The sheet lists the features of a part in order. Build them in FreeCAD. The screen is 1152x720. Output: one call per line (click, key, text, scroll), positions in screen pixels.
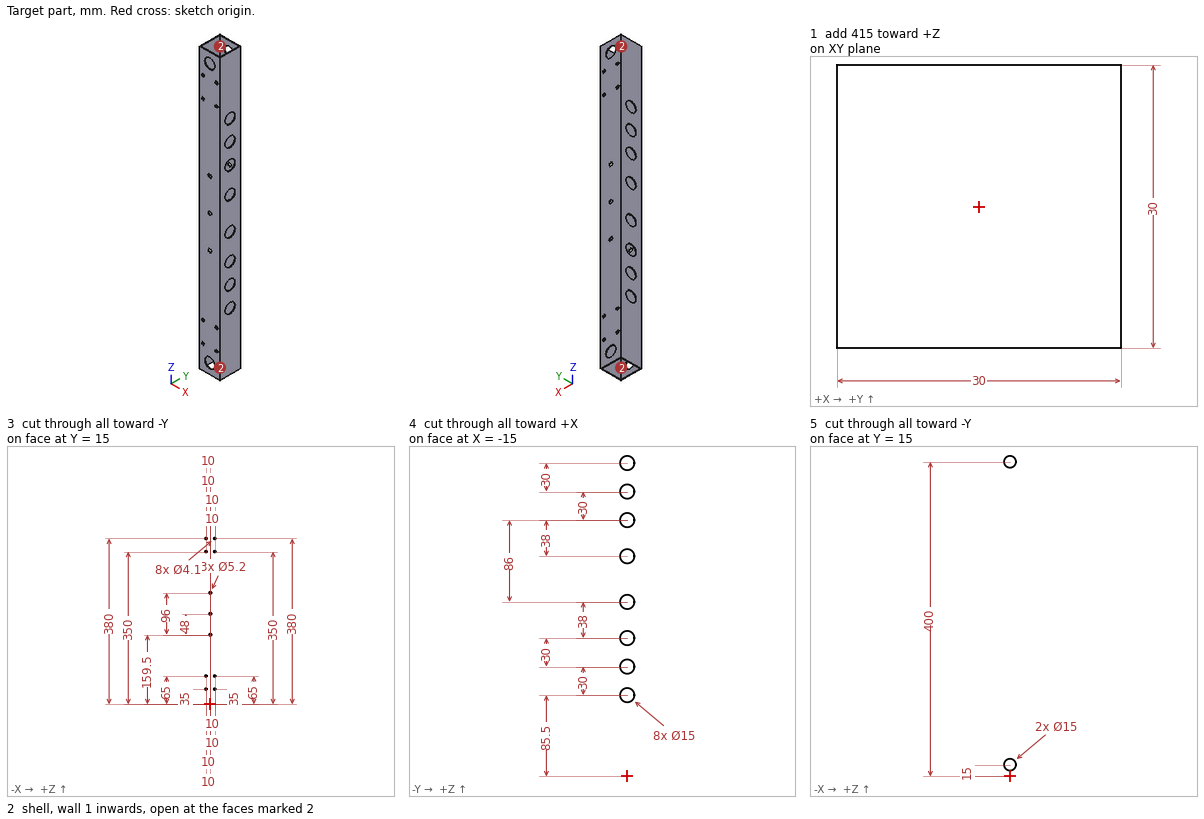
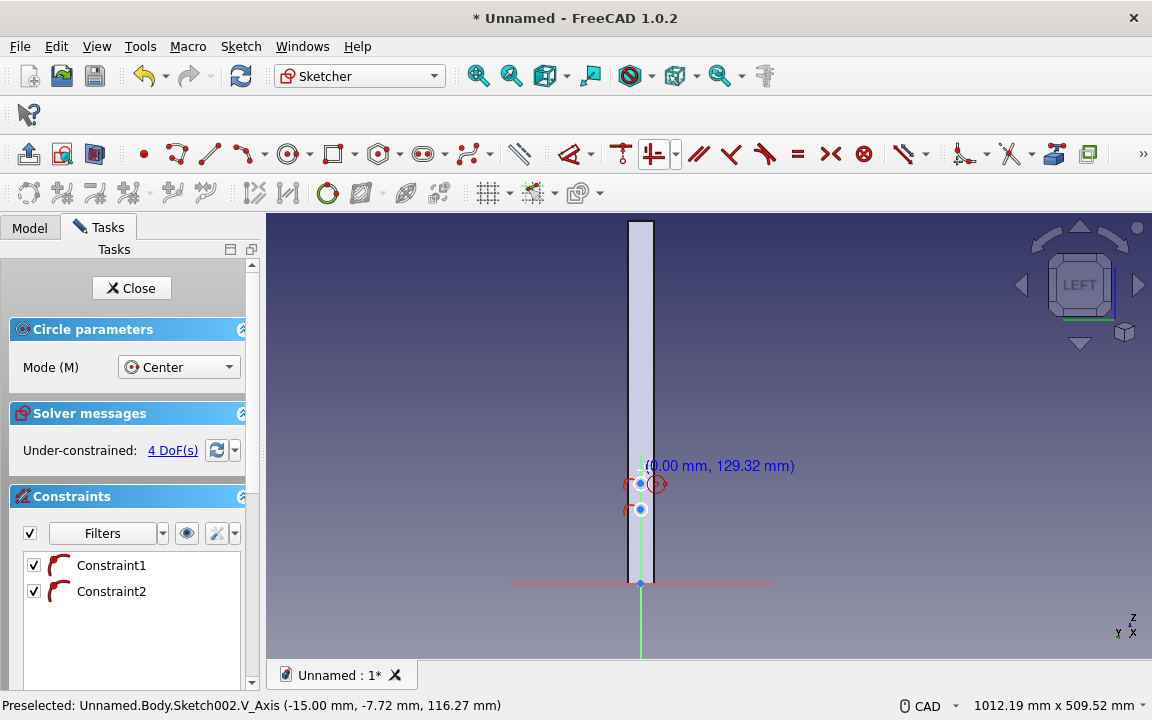
click(641, 457)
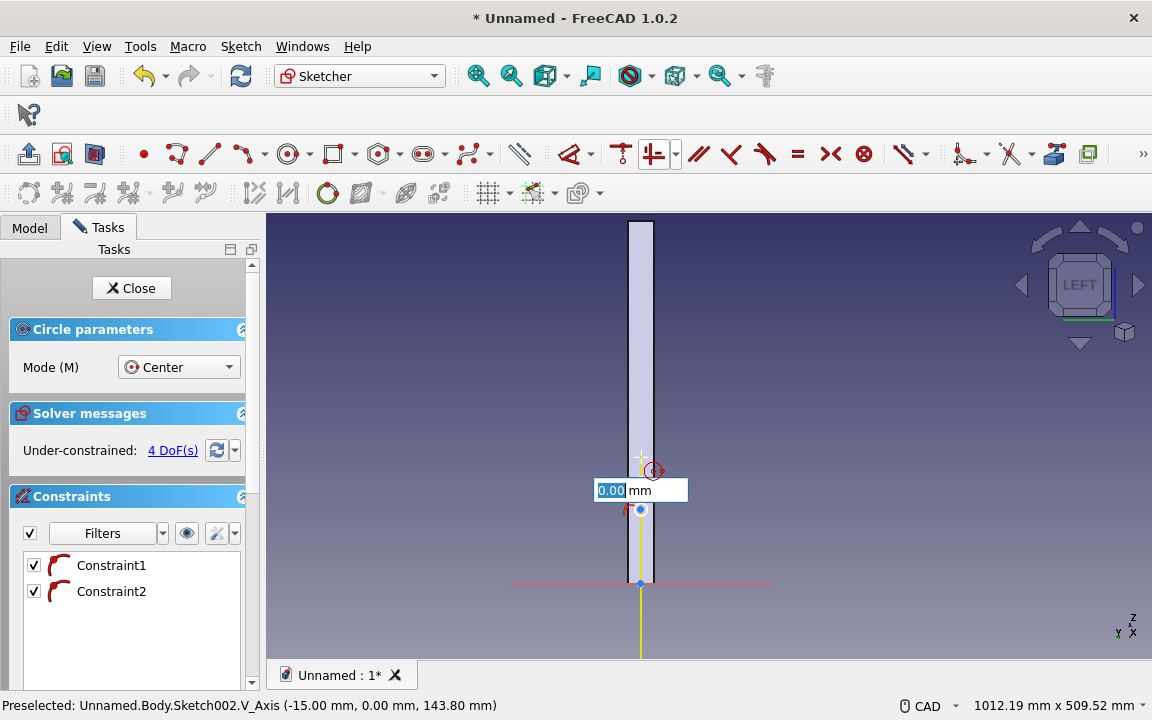
scroll(647, 454, up, 5)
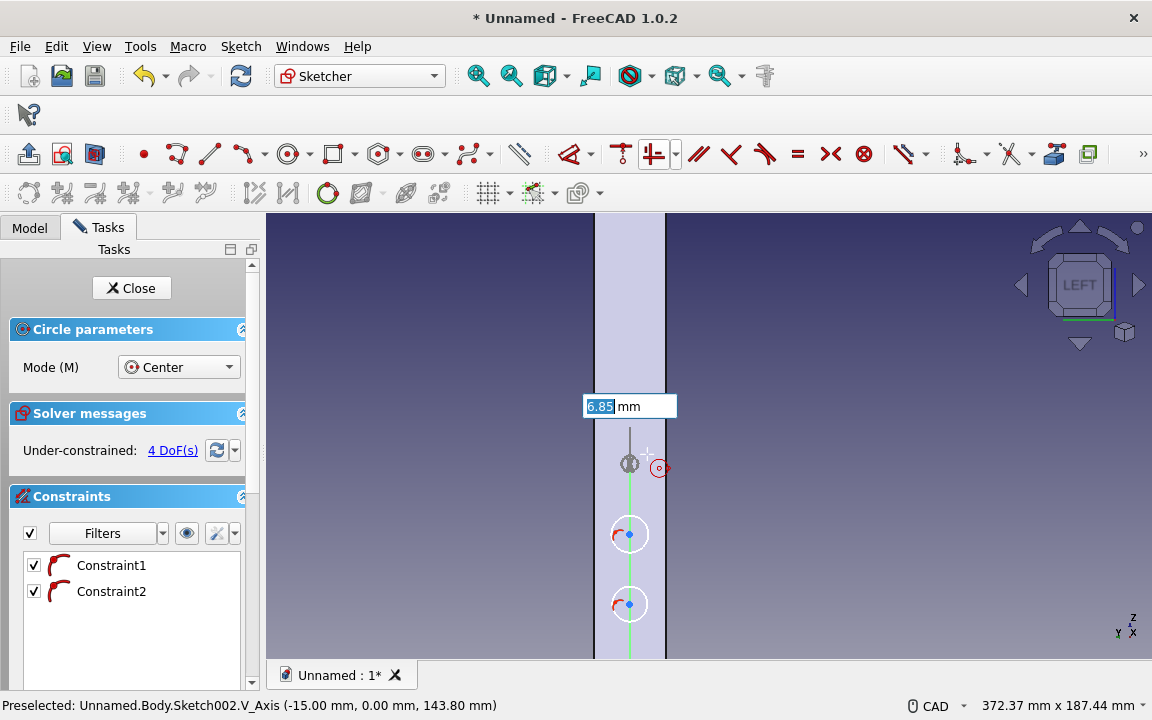
click(647, 454)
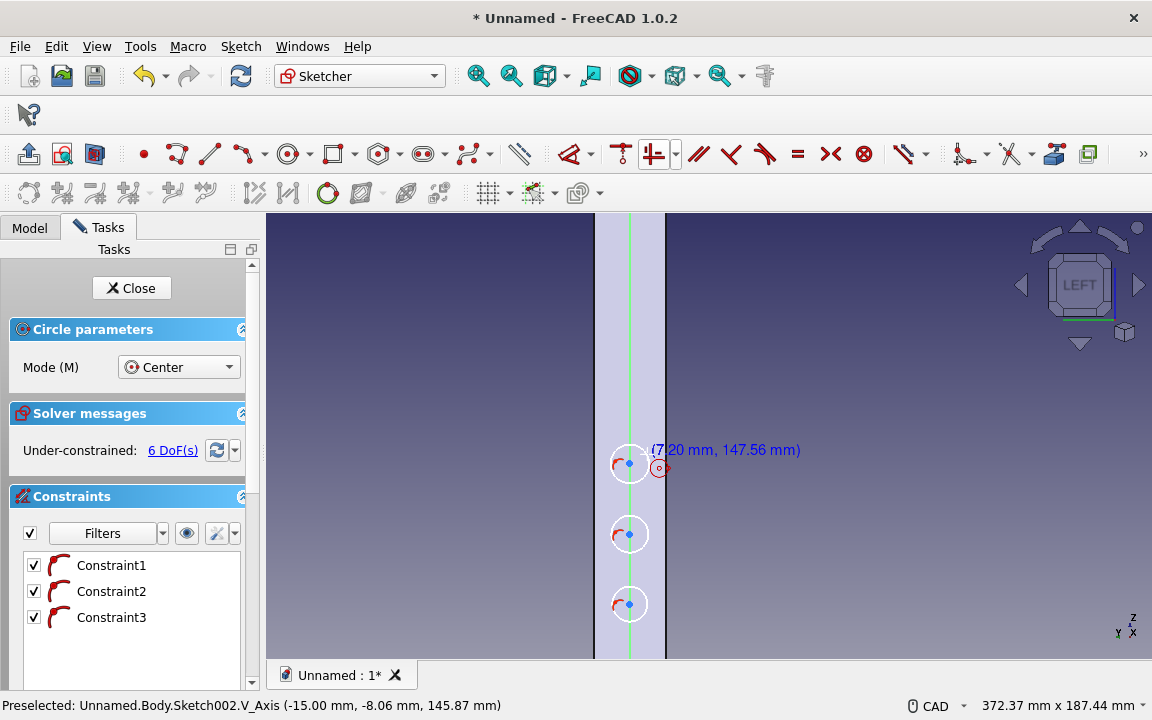
scroll(647, 454, down, 5)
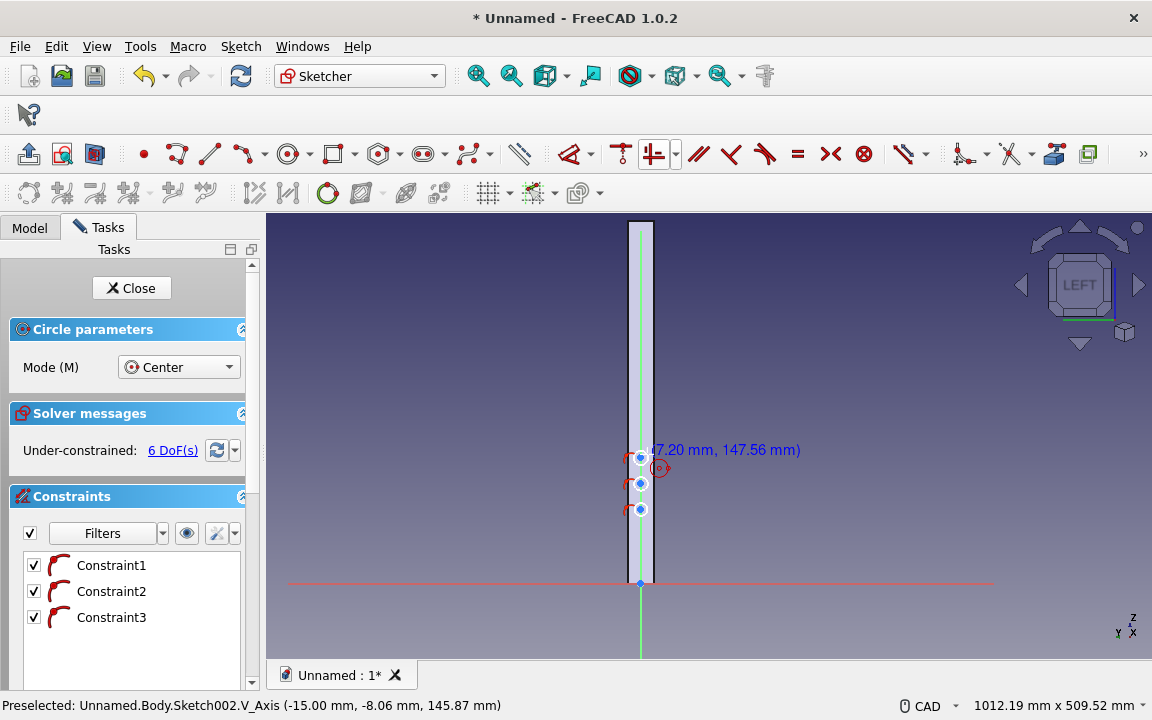
scroll(641, 348, up, 7)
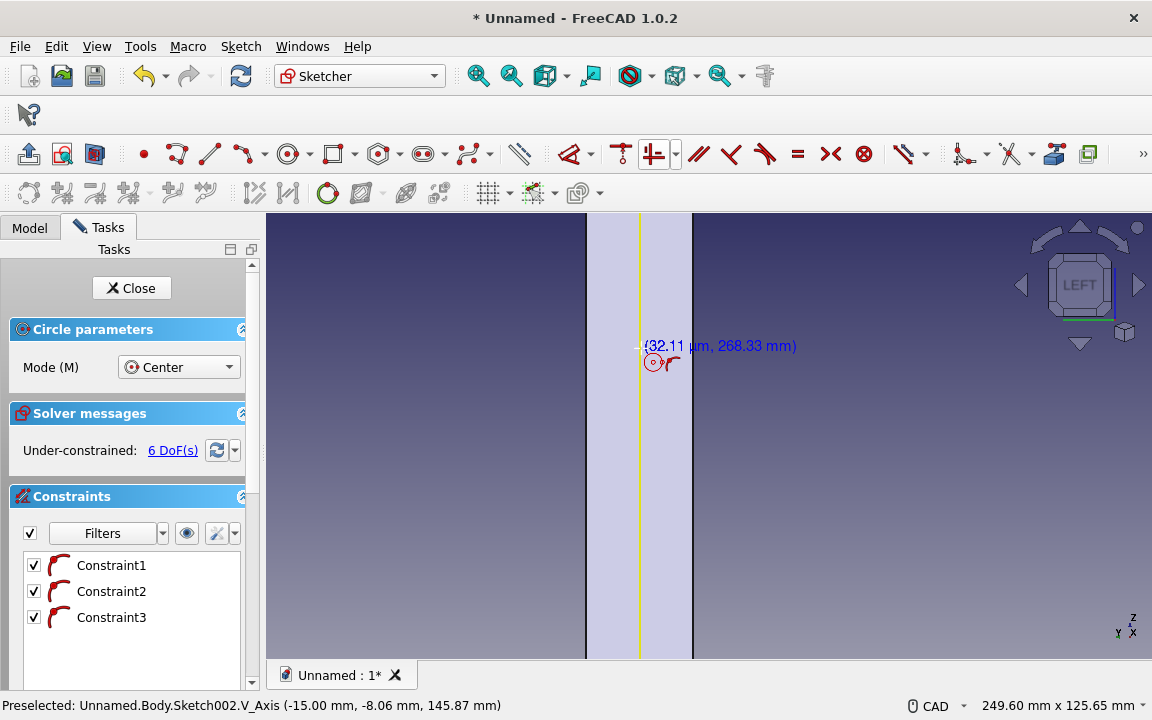
scroll(641, 348, down, 7)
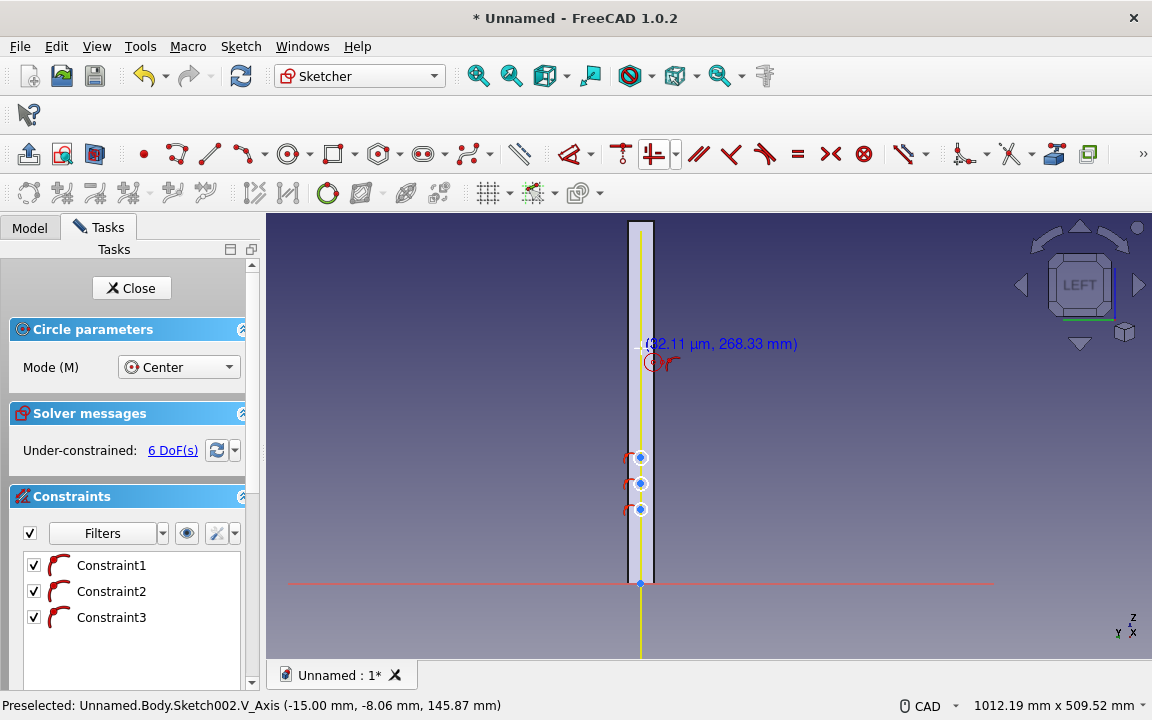
click(641, 348)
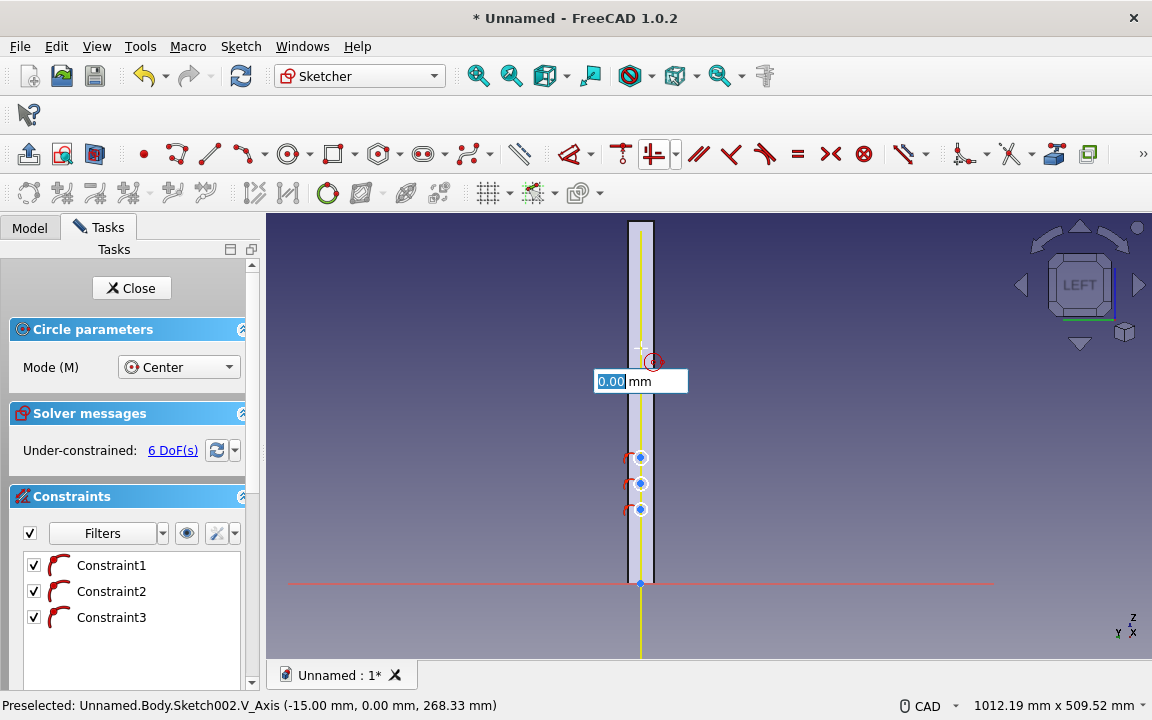
scroll(647, 346, up, 5)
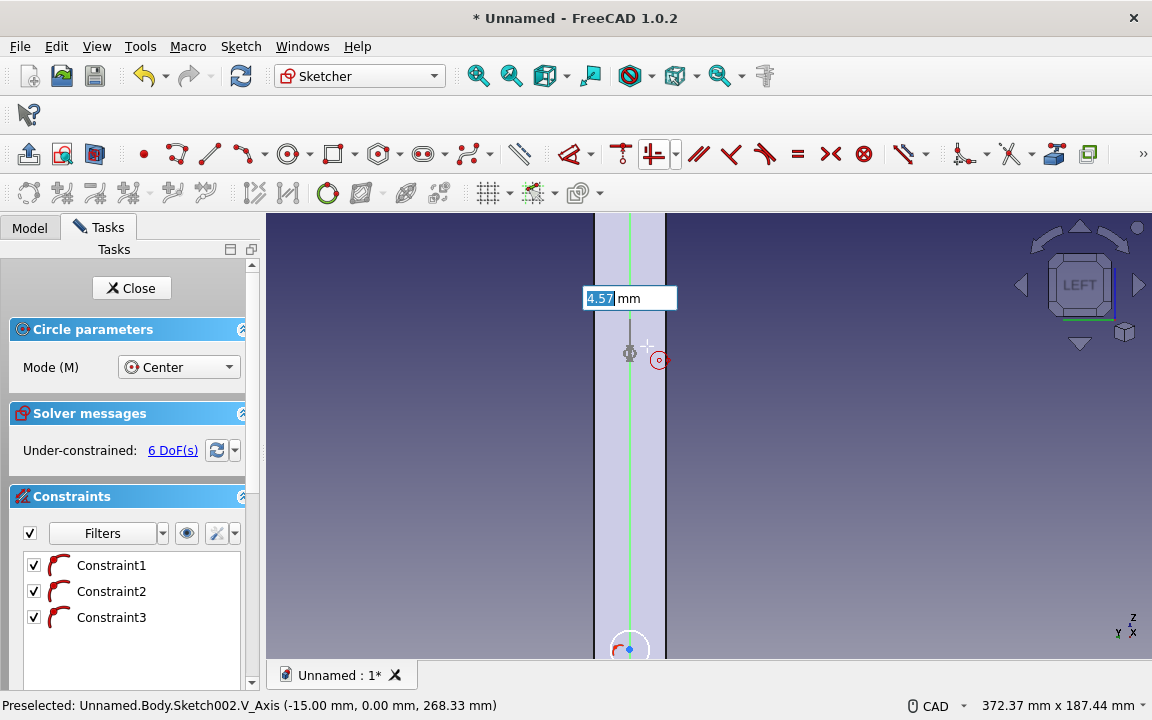
click(647, 345)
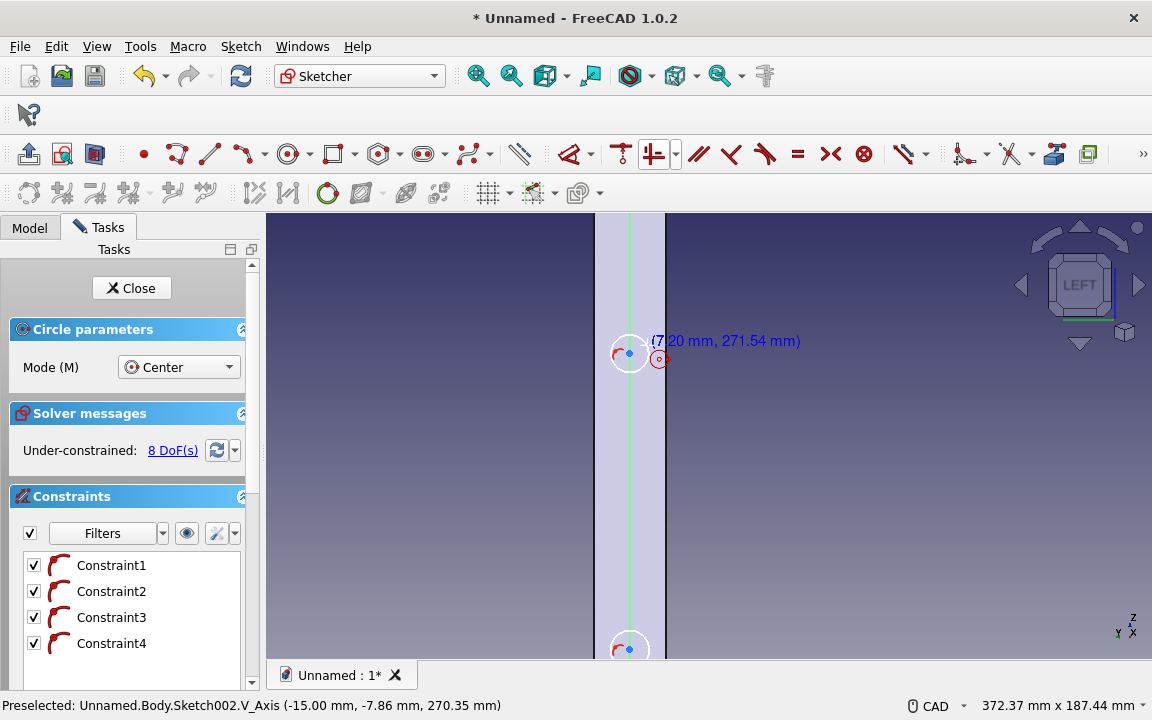
scroll(630, 279, up, 2)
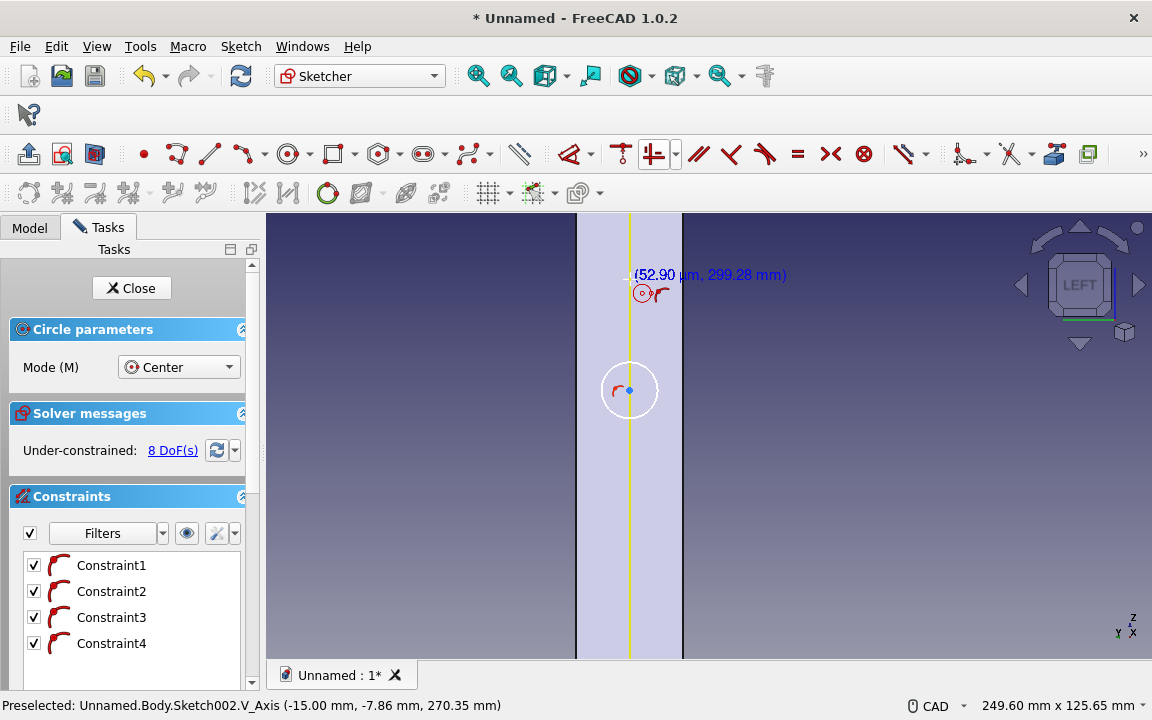
scroll(644, 335, down, 7)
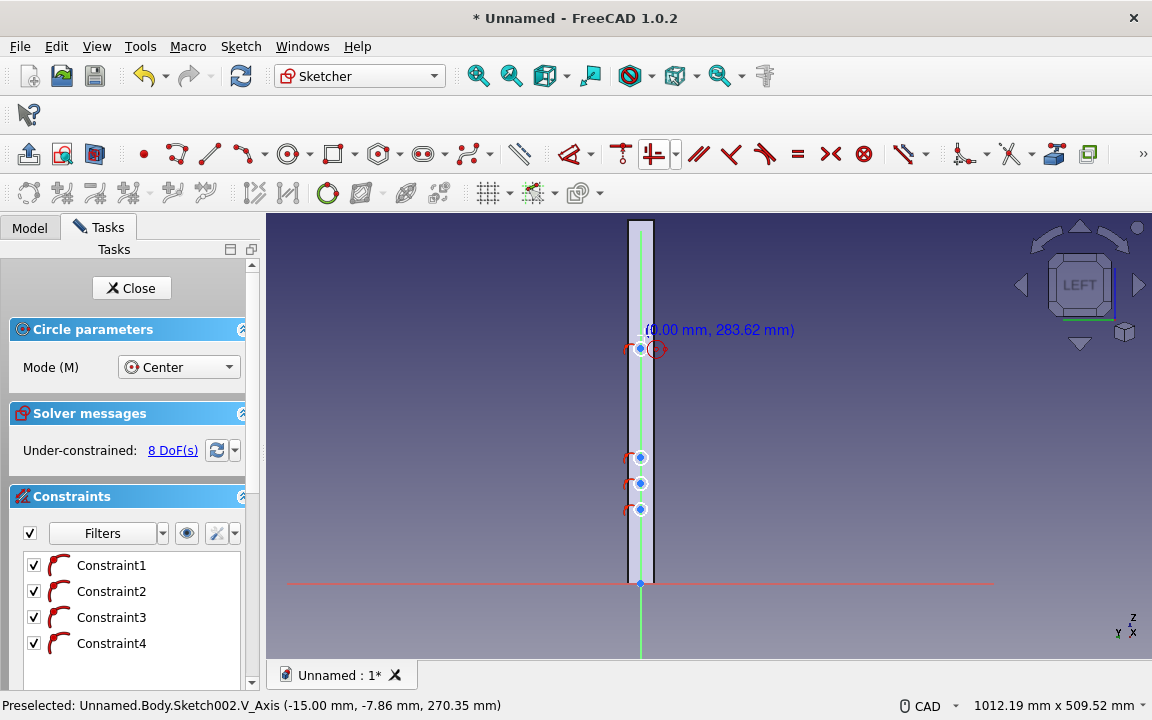
click(641, 322)